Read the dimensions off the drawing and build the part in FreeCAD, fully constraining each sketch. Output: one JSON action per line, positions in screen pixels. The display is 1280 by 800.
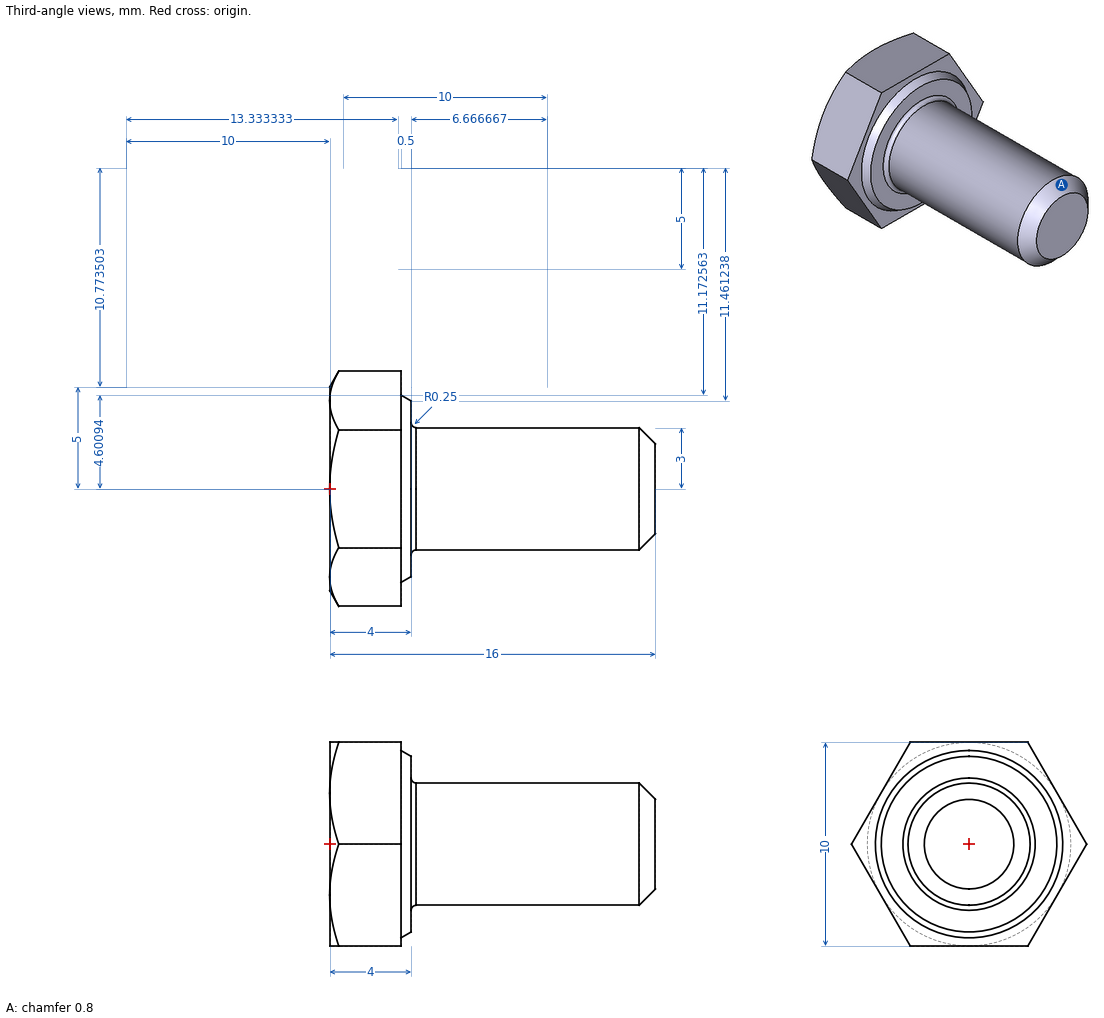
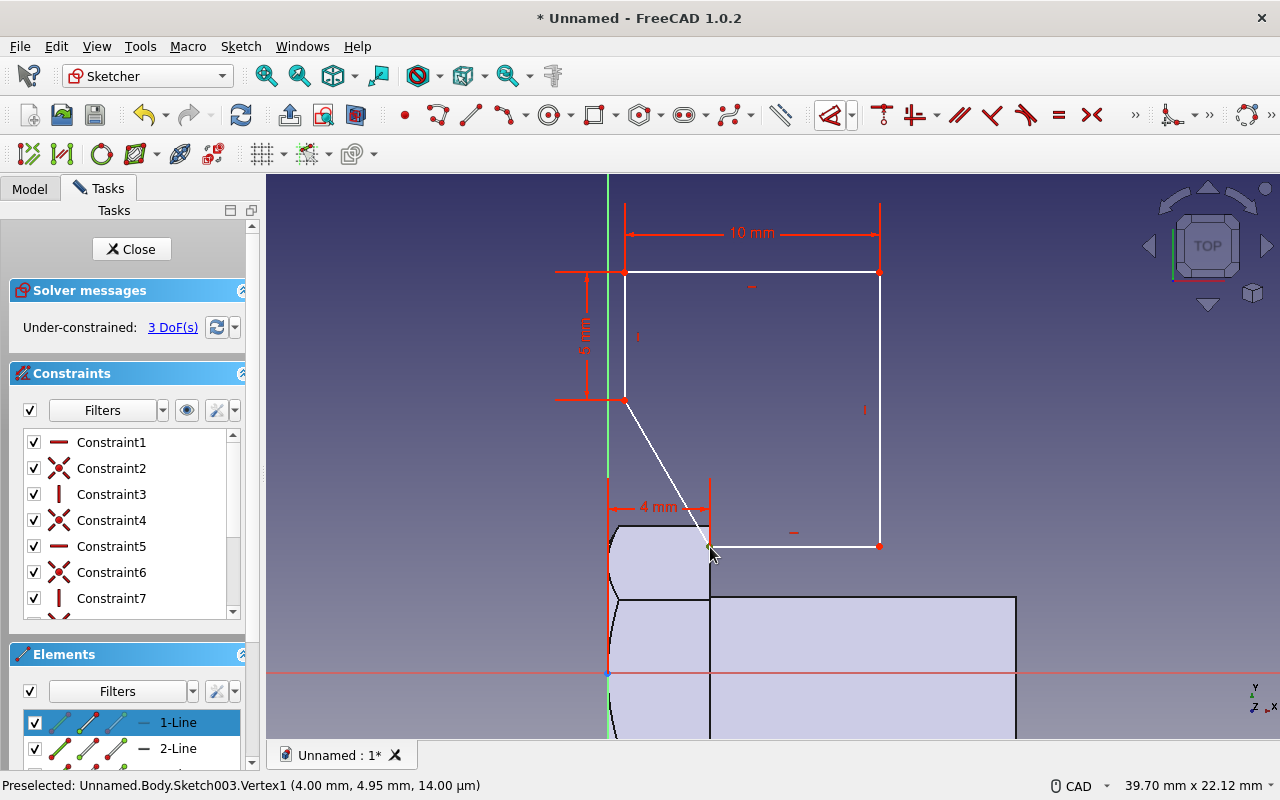
{"action": "left_click", "coordinate": [852, 116]}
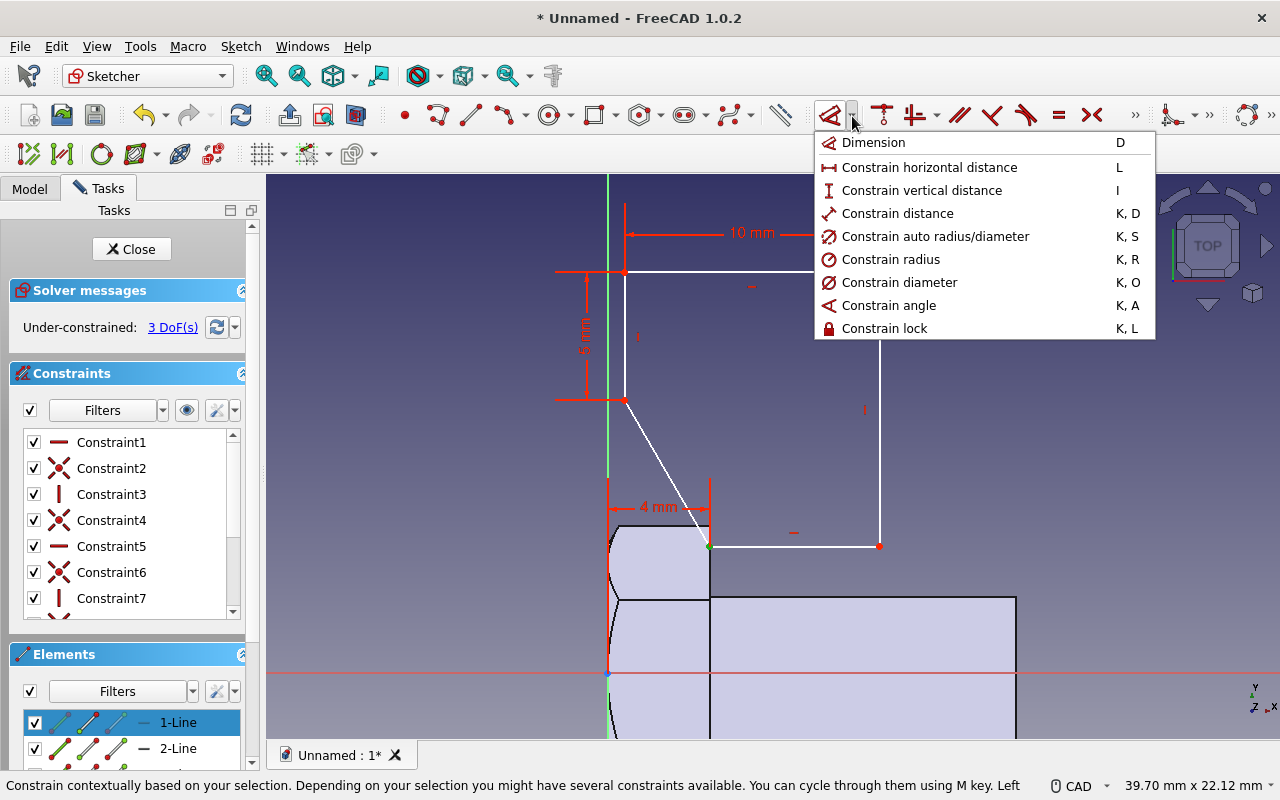
{"action": "left_click", "coordinate": [985, 190]}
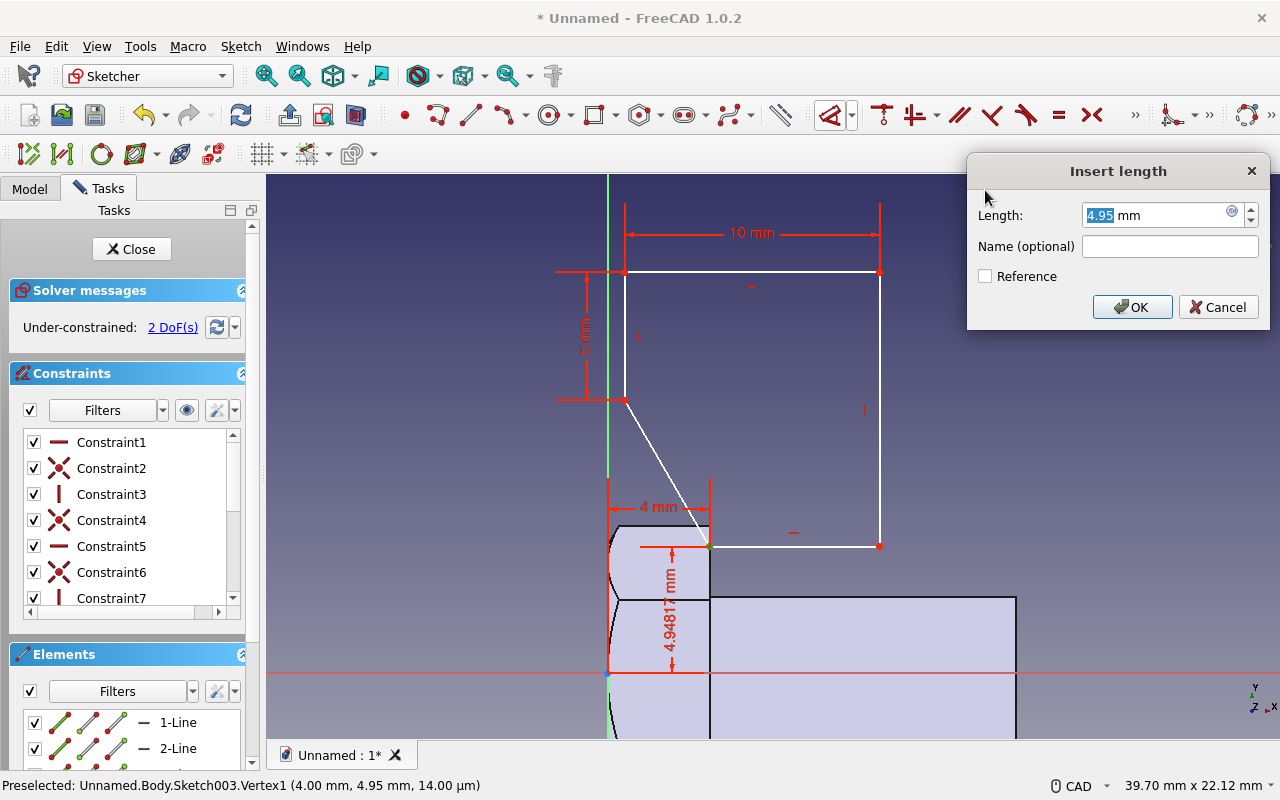
{"action": "type", "text": "5"}
{"action": "key", "text": "Return"}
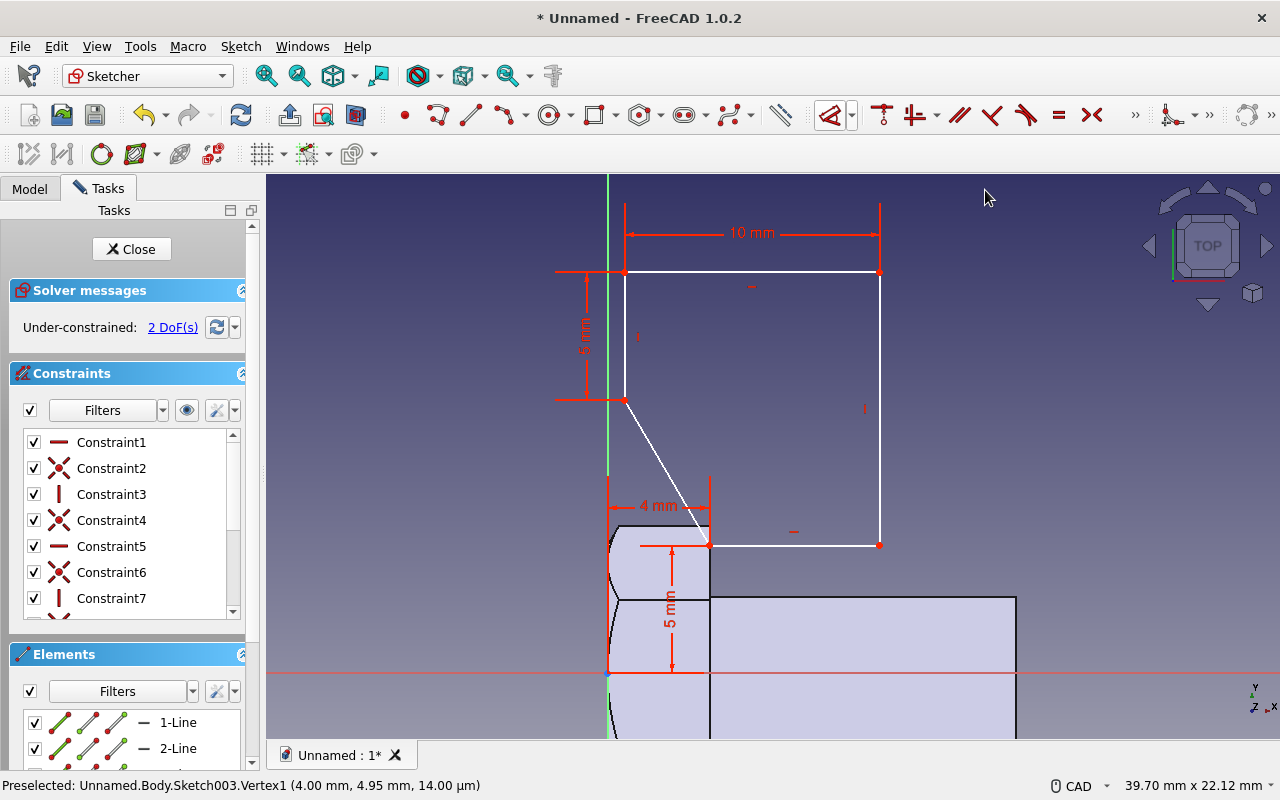
{"action": "left_click", "coordinate": [761, 546]}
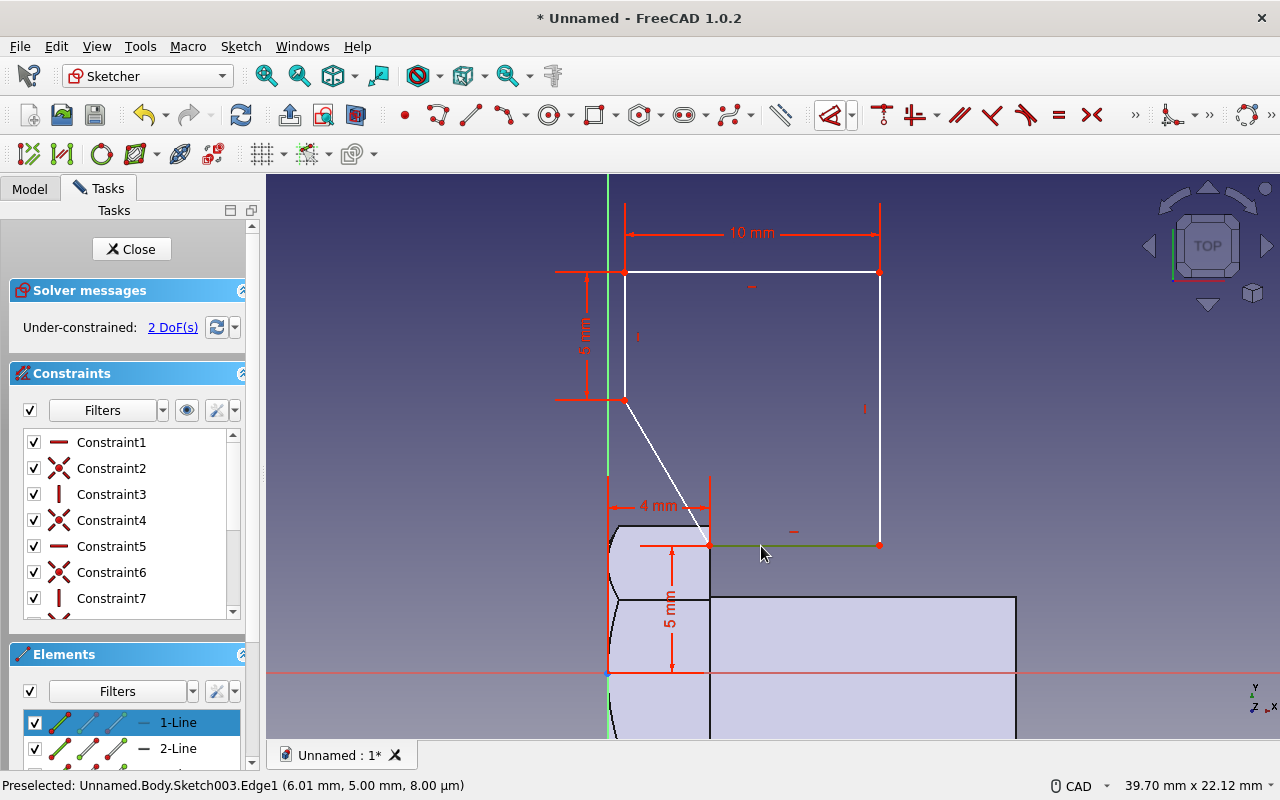
{"action": "key", "text": "l"}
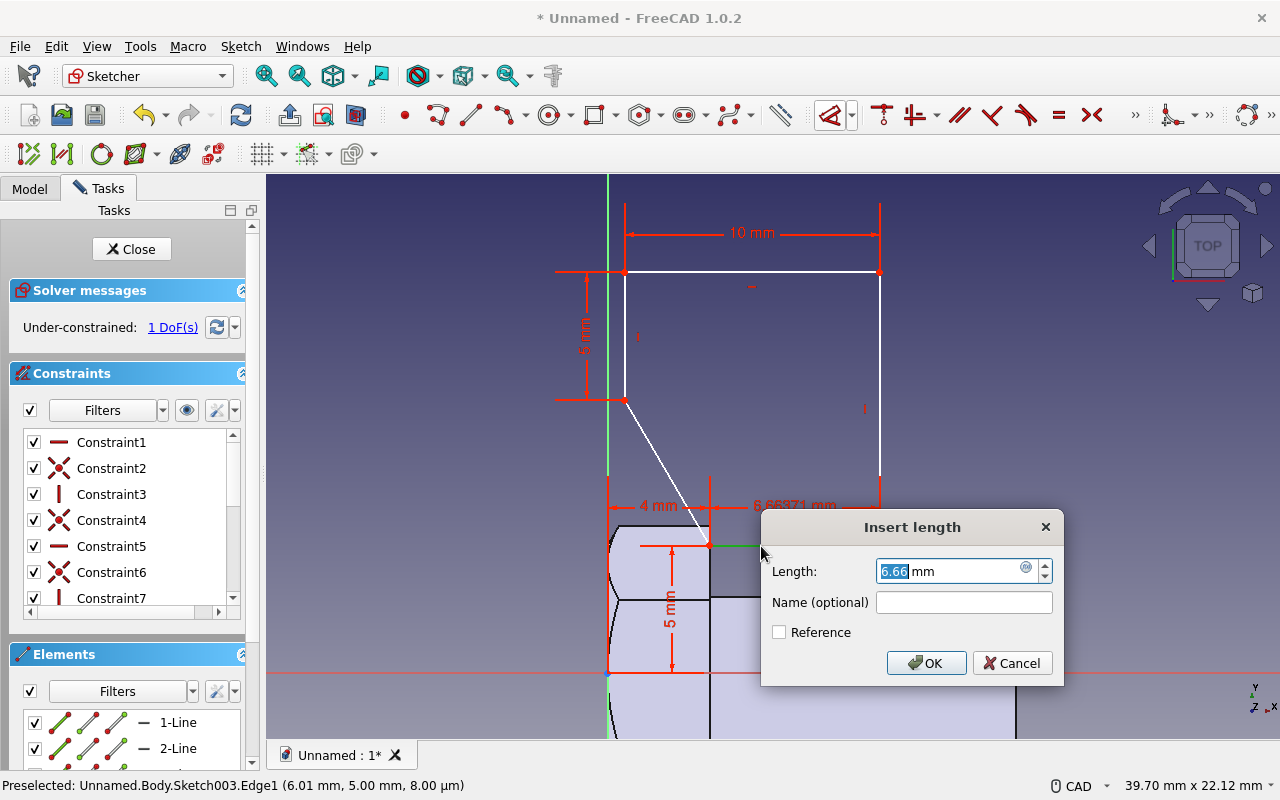
{"action": "type", "text": "6.666667"}
{"action": "key", "text": "Return"}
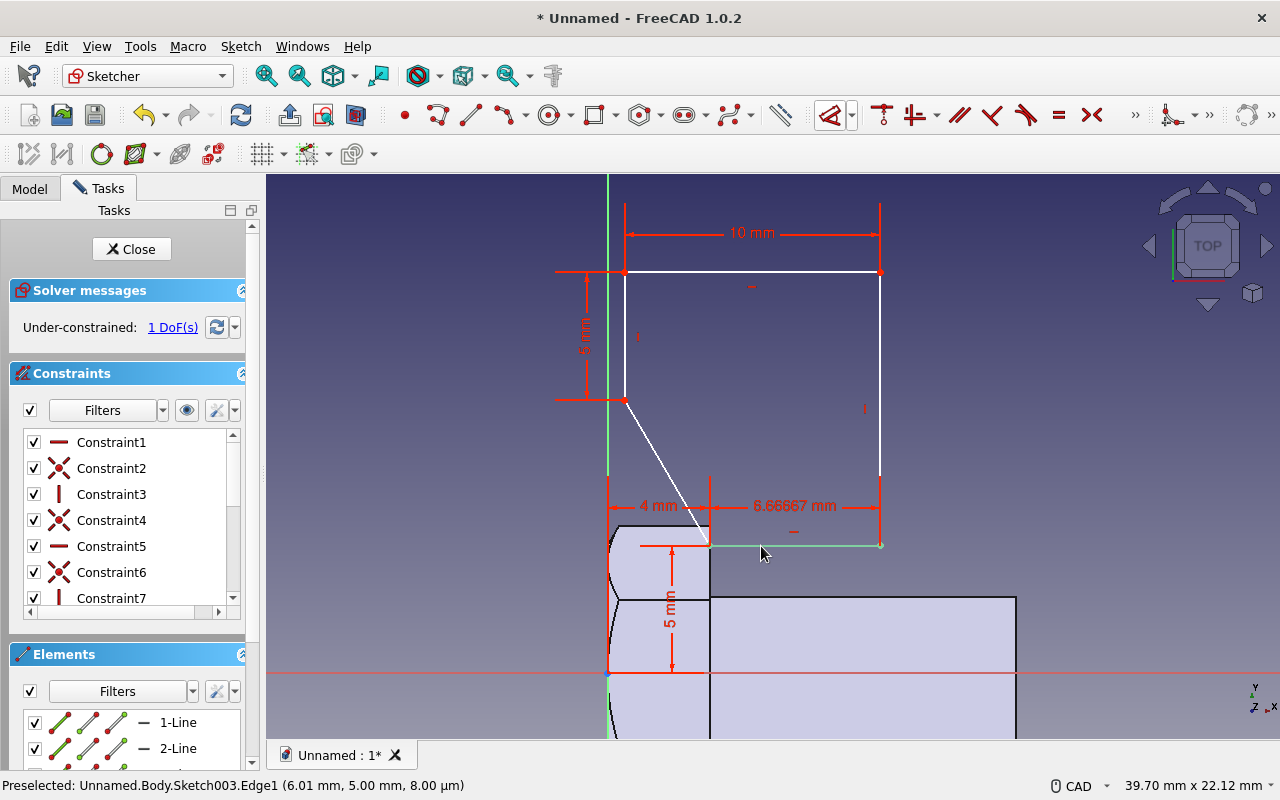
{"action": "left_click", "coordinate": [880, 464]}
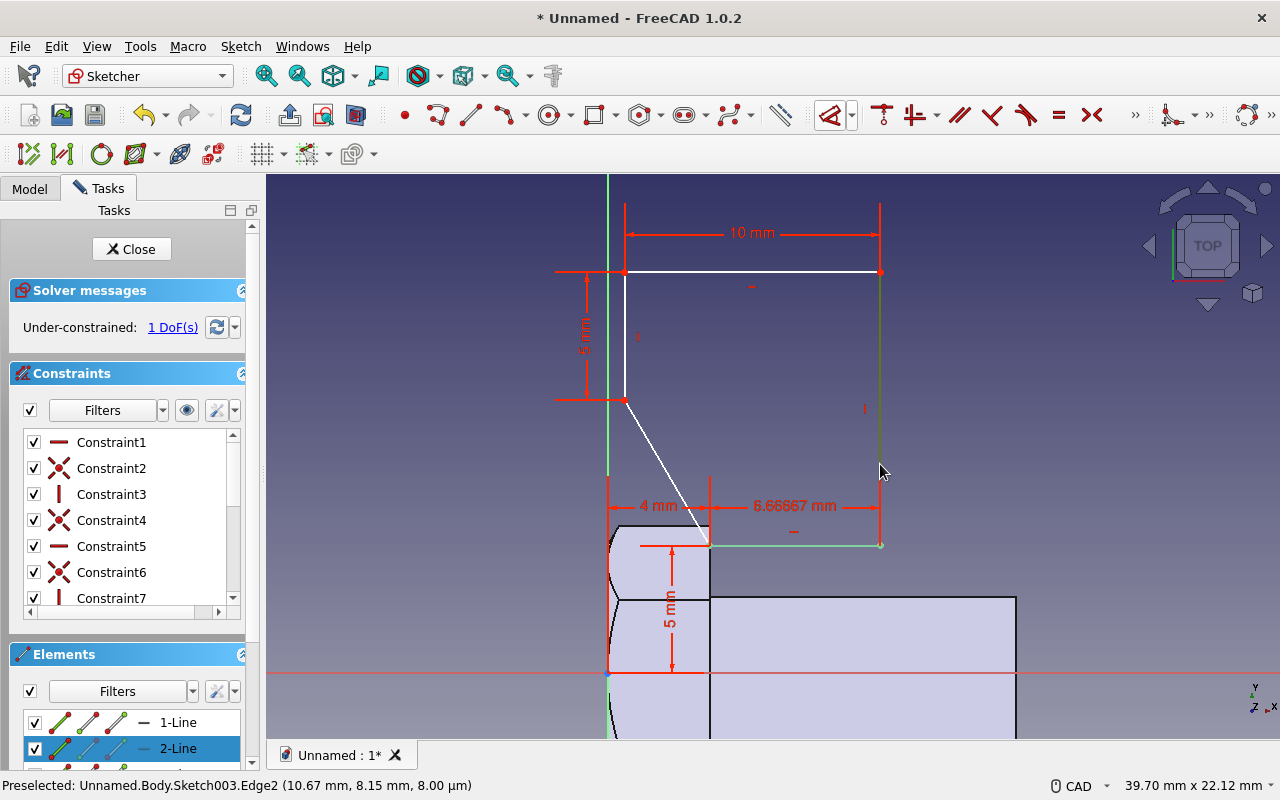
{"action": "key", "text": "i"}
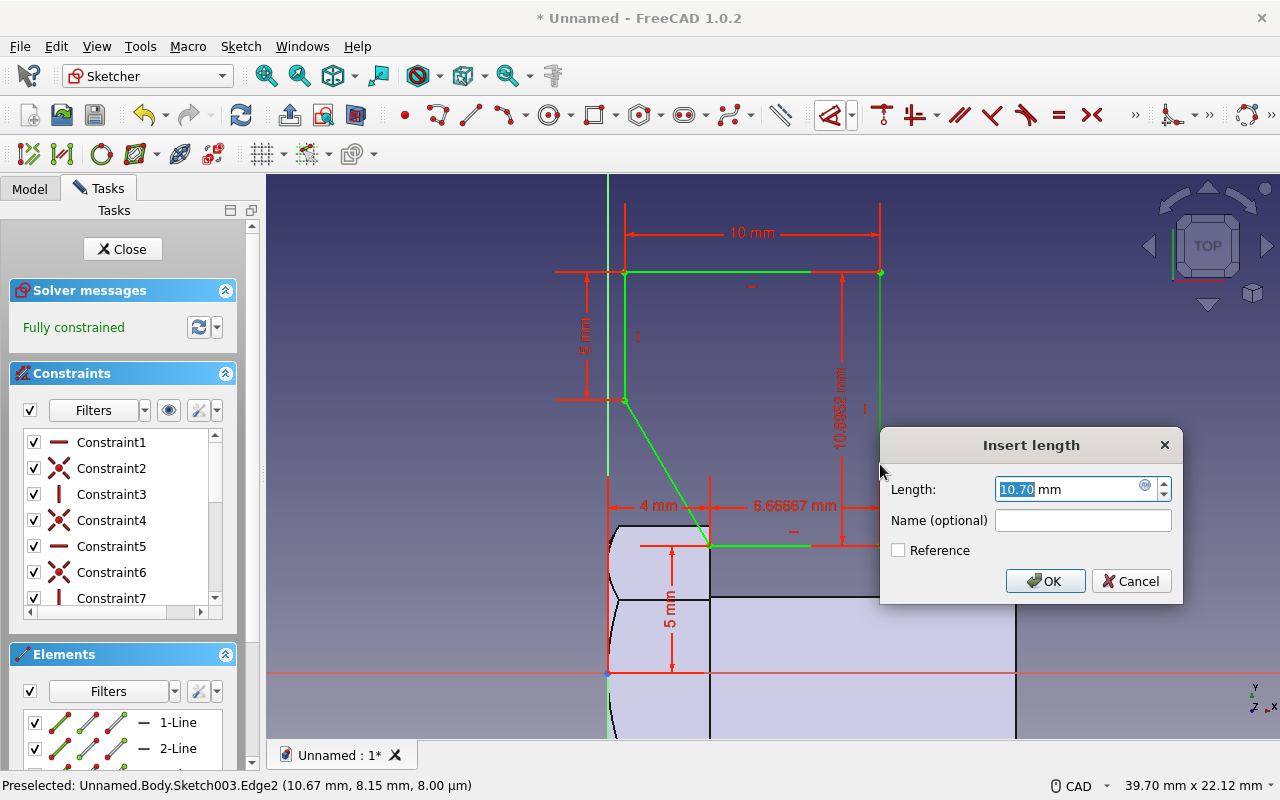
{"action": "type", "text": "10.773503"}
{"action": "key", "text": "Return"}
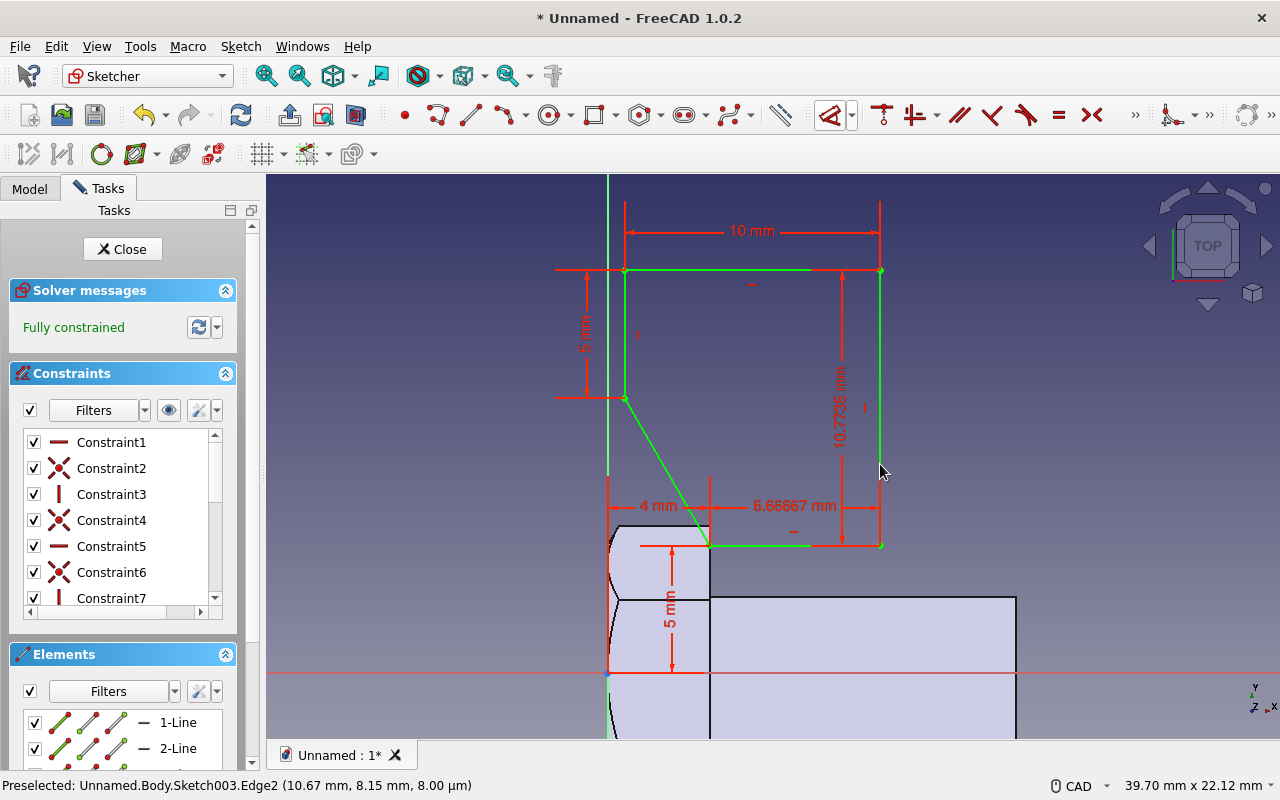
{"action": "left_click", "coordinate": [123, 249]}